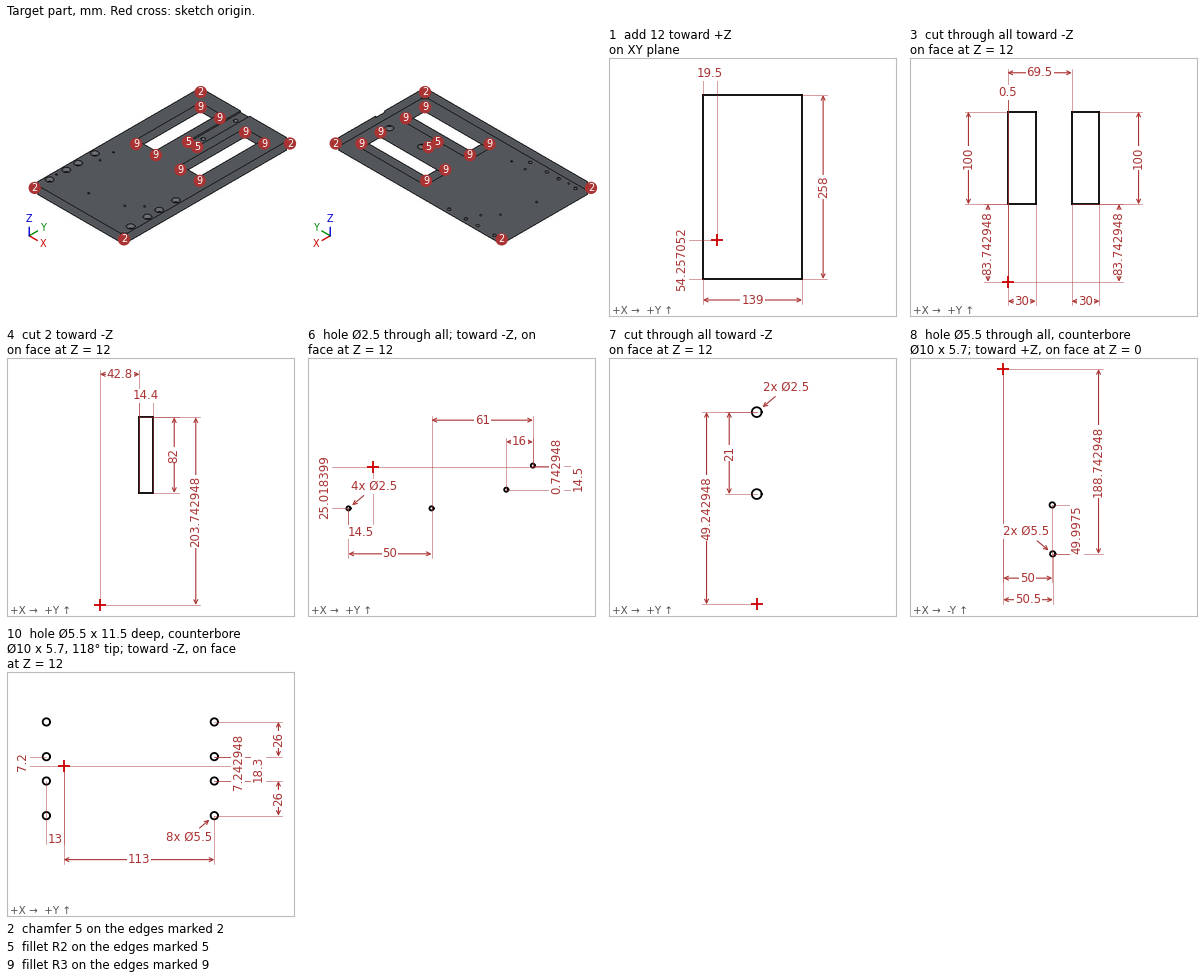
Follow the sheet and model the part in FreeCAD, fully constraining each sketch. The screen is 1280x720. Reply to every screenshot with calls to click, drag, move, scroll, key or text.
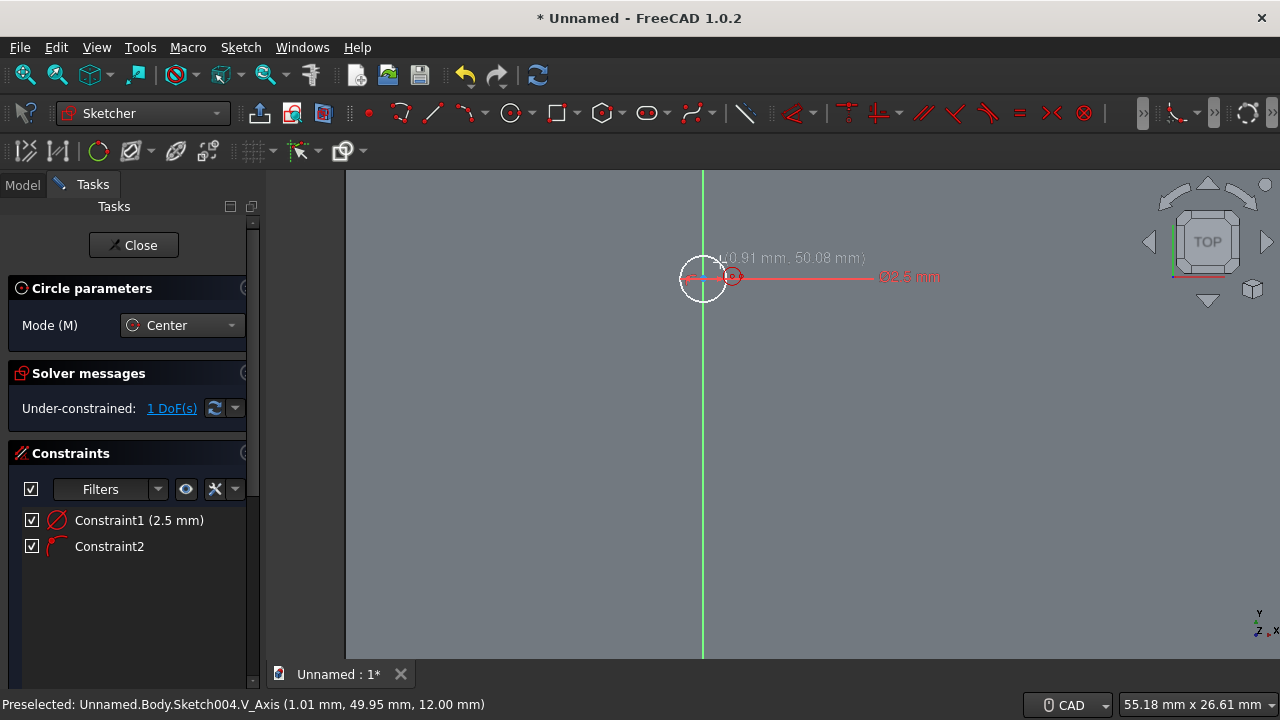
scroll(705, 283, down, 6)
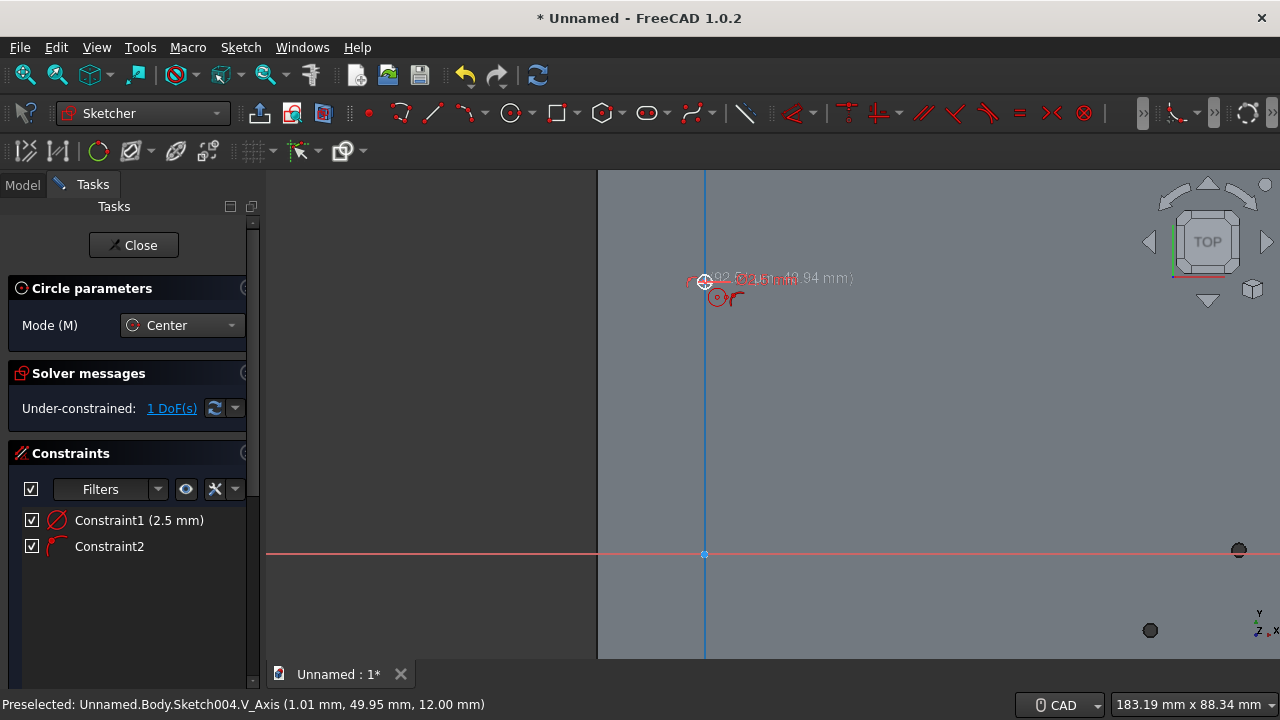
scroll(705, 398, up, 6)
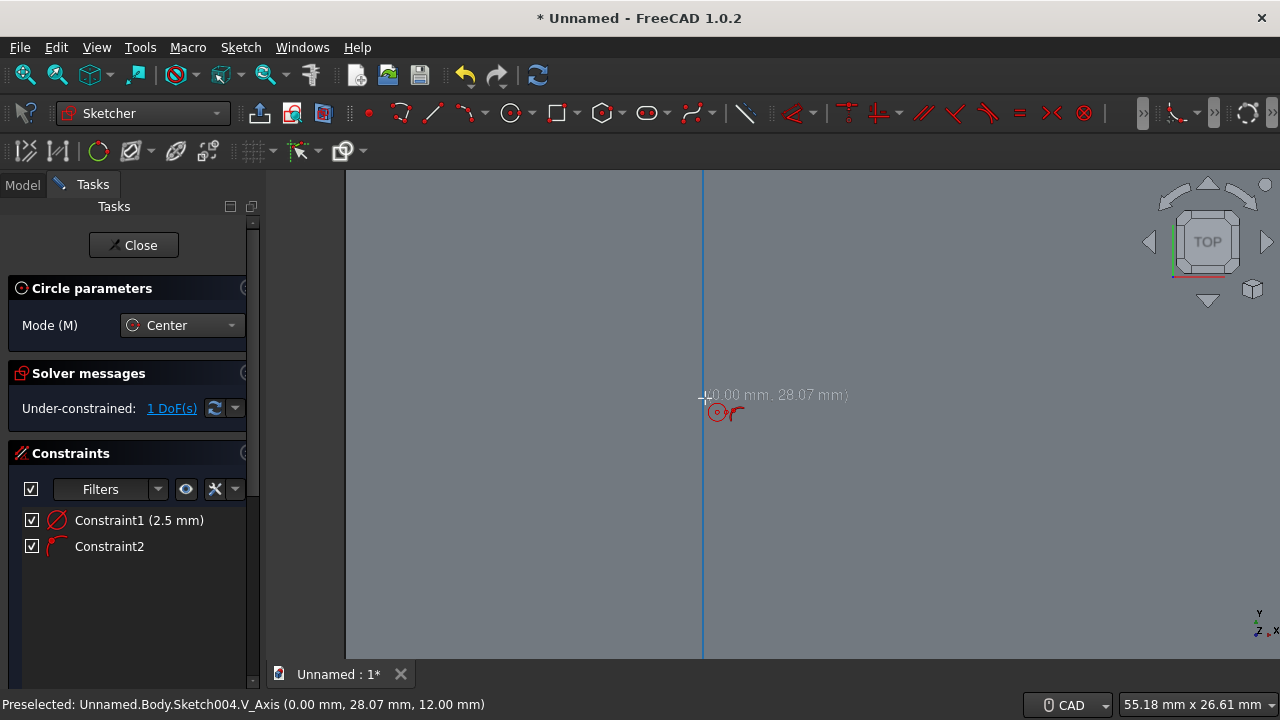
click(703, 397)
move(720, 381)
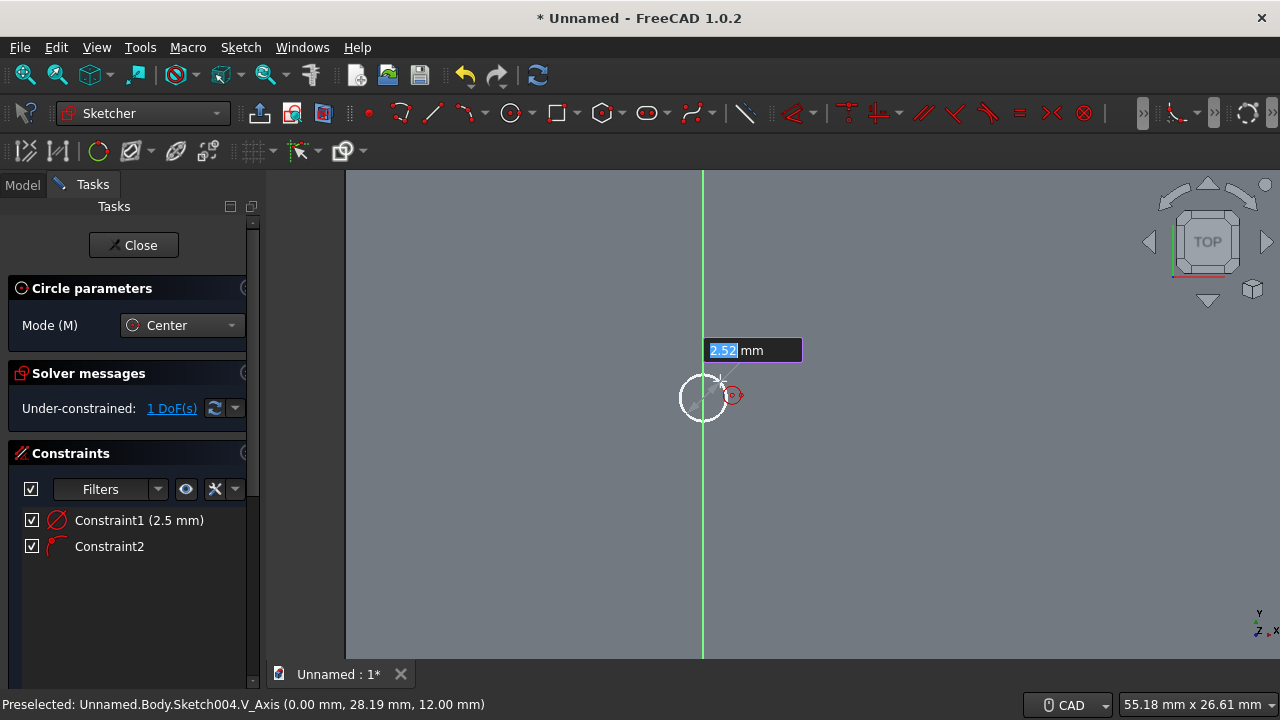
text(2.5)
key(Return)
key(Escape)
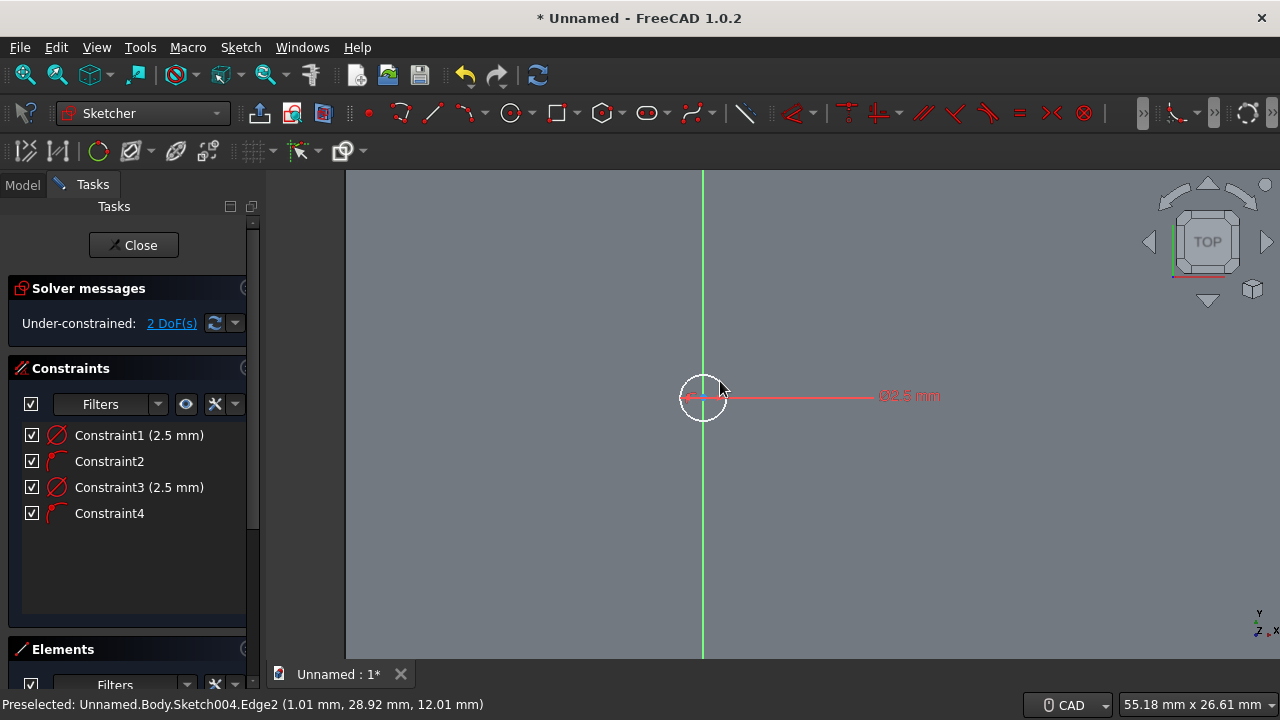
click(792, 114)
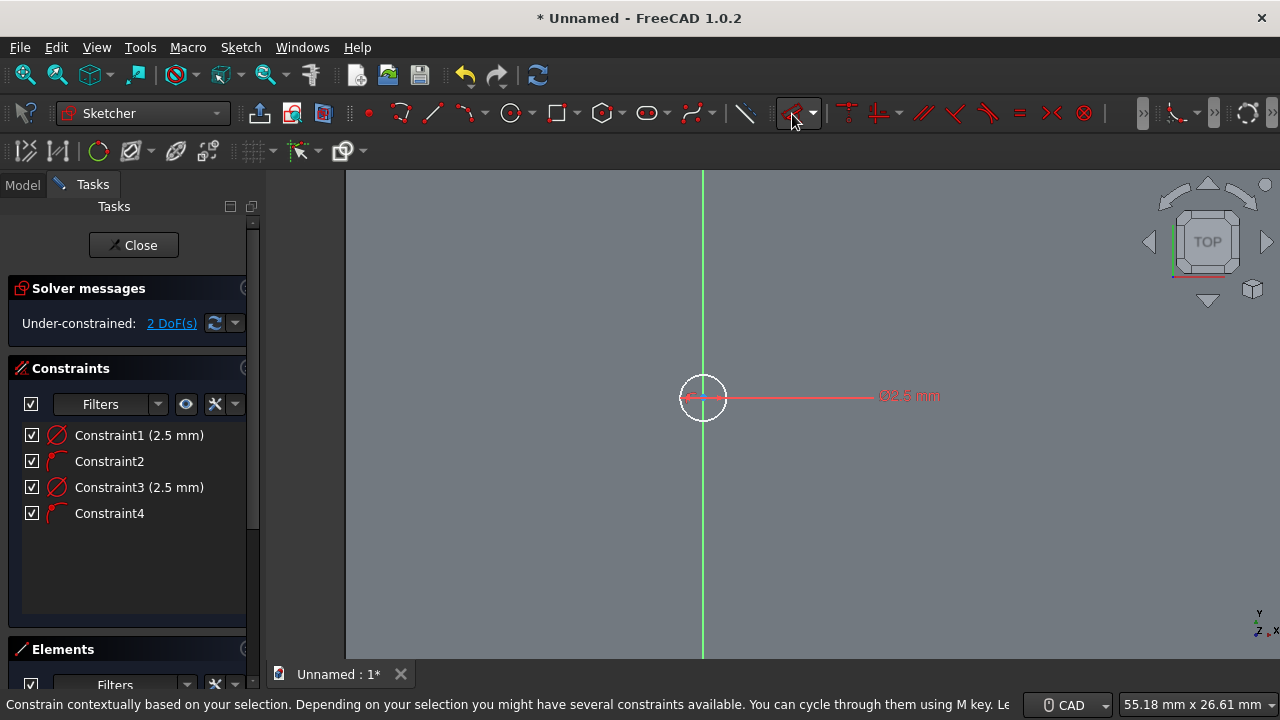
scroll(705, 398, down, 6)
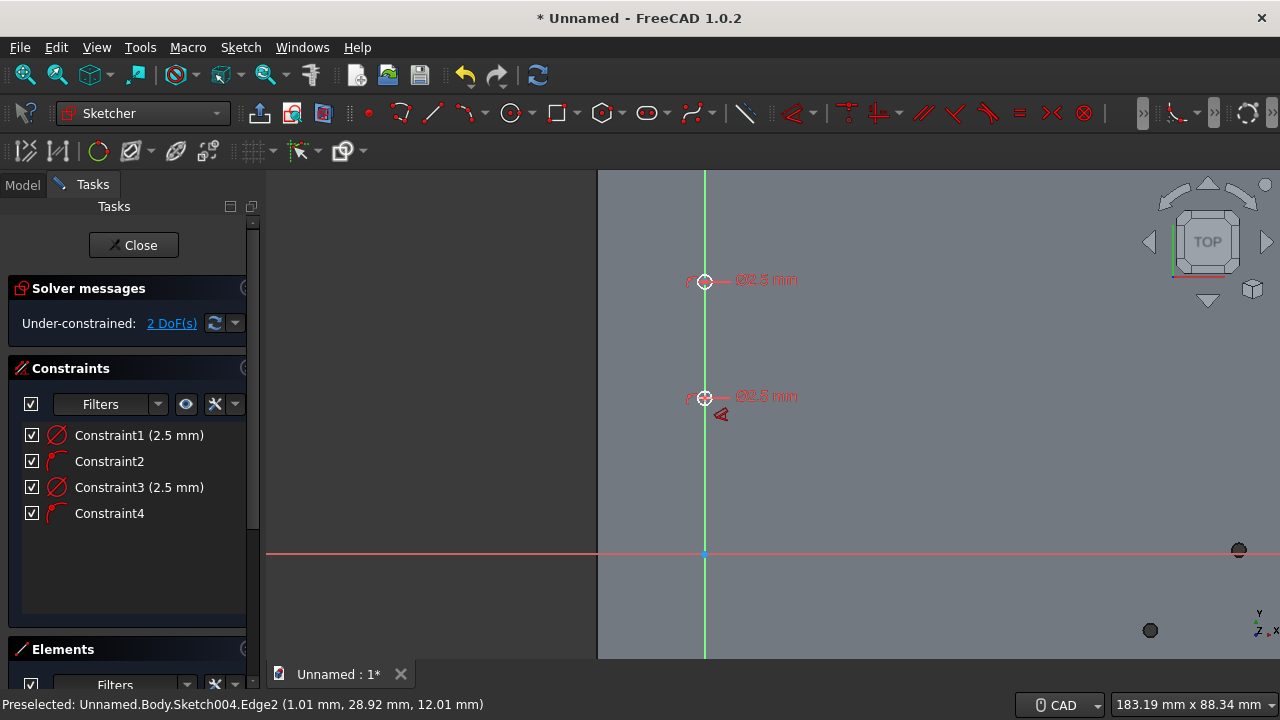
click(705, 282)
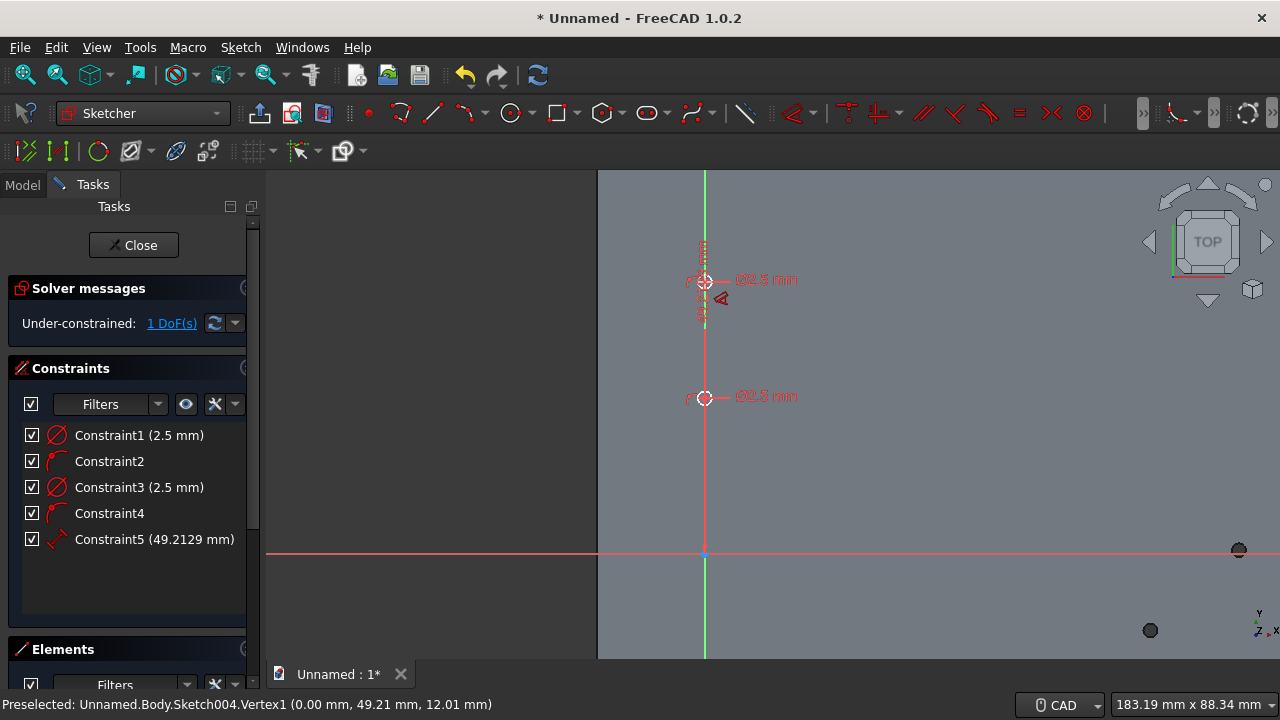
click(705, 398)
click(739, 340)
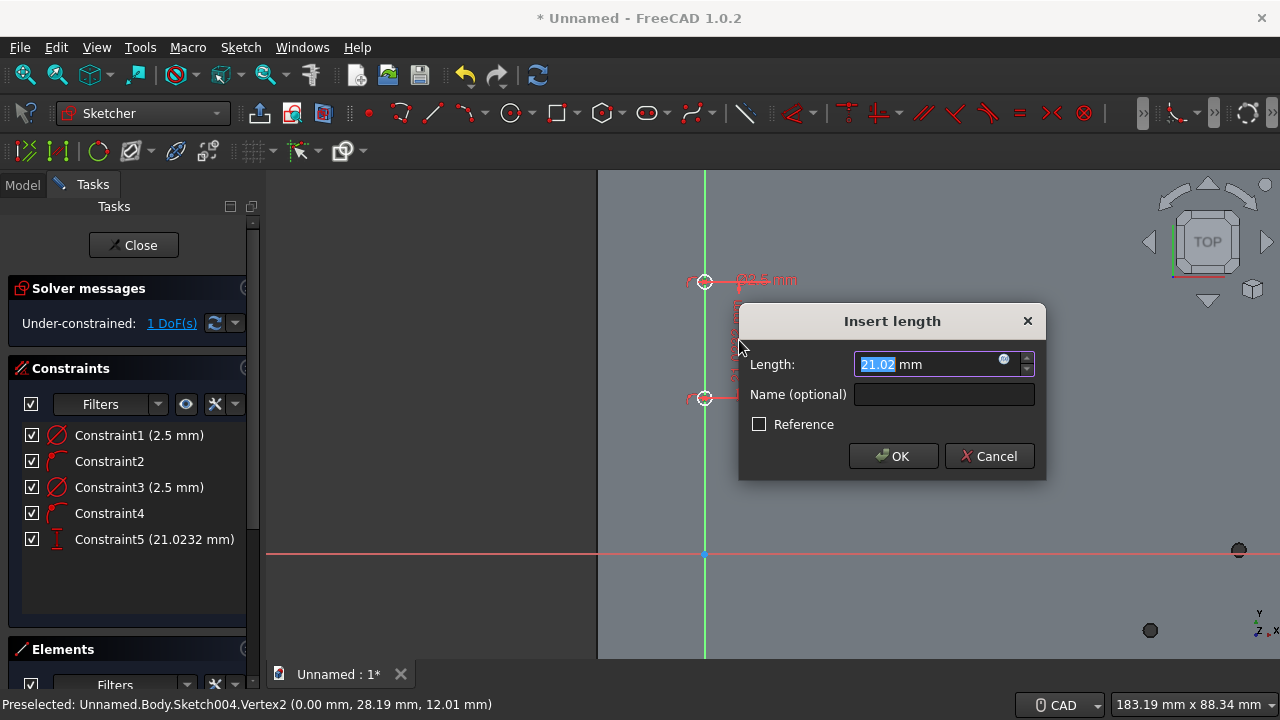
text(21)
key(Return)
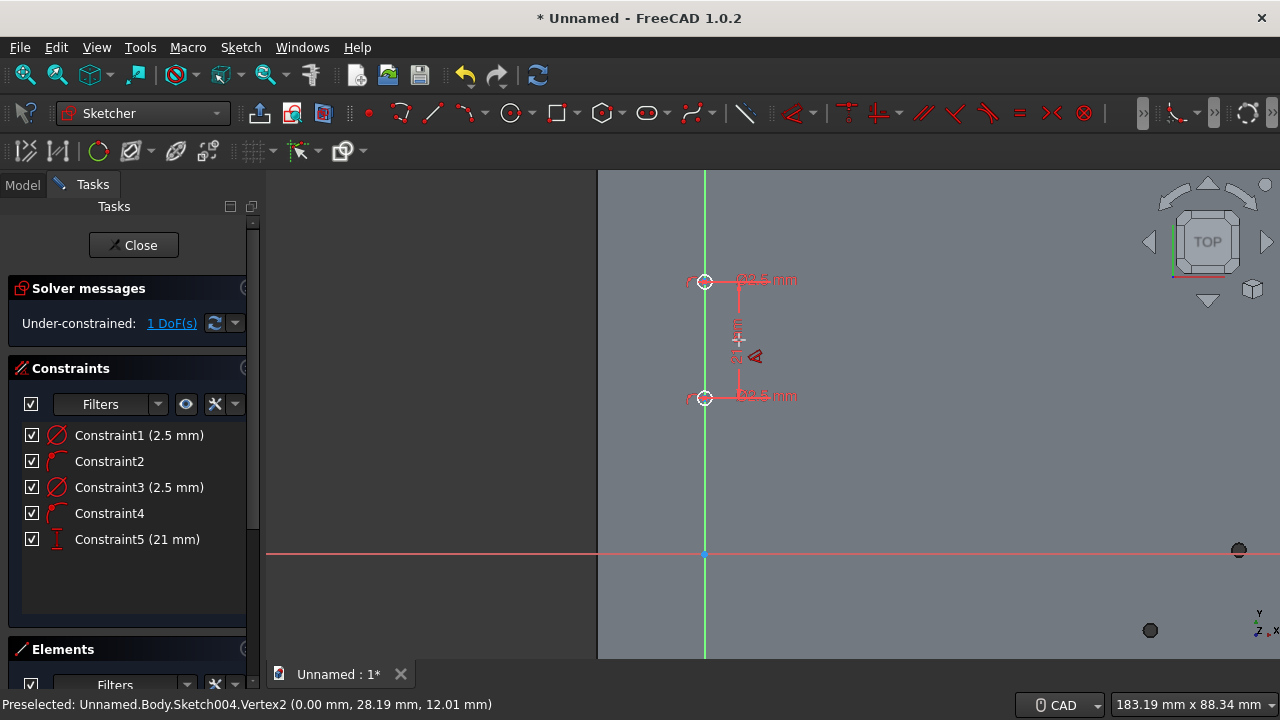
click(705, 282)
click(739, 418)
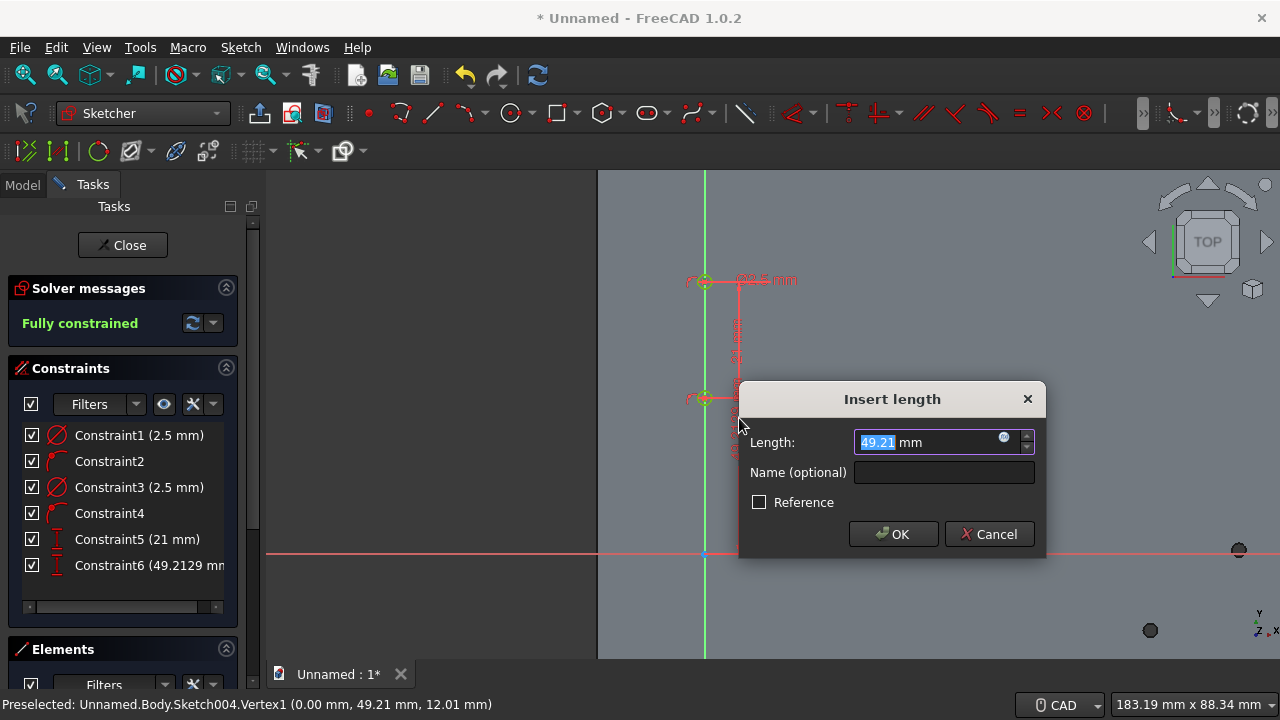
text(49.242948)
key(Return)
key(Escape)